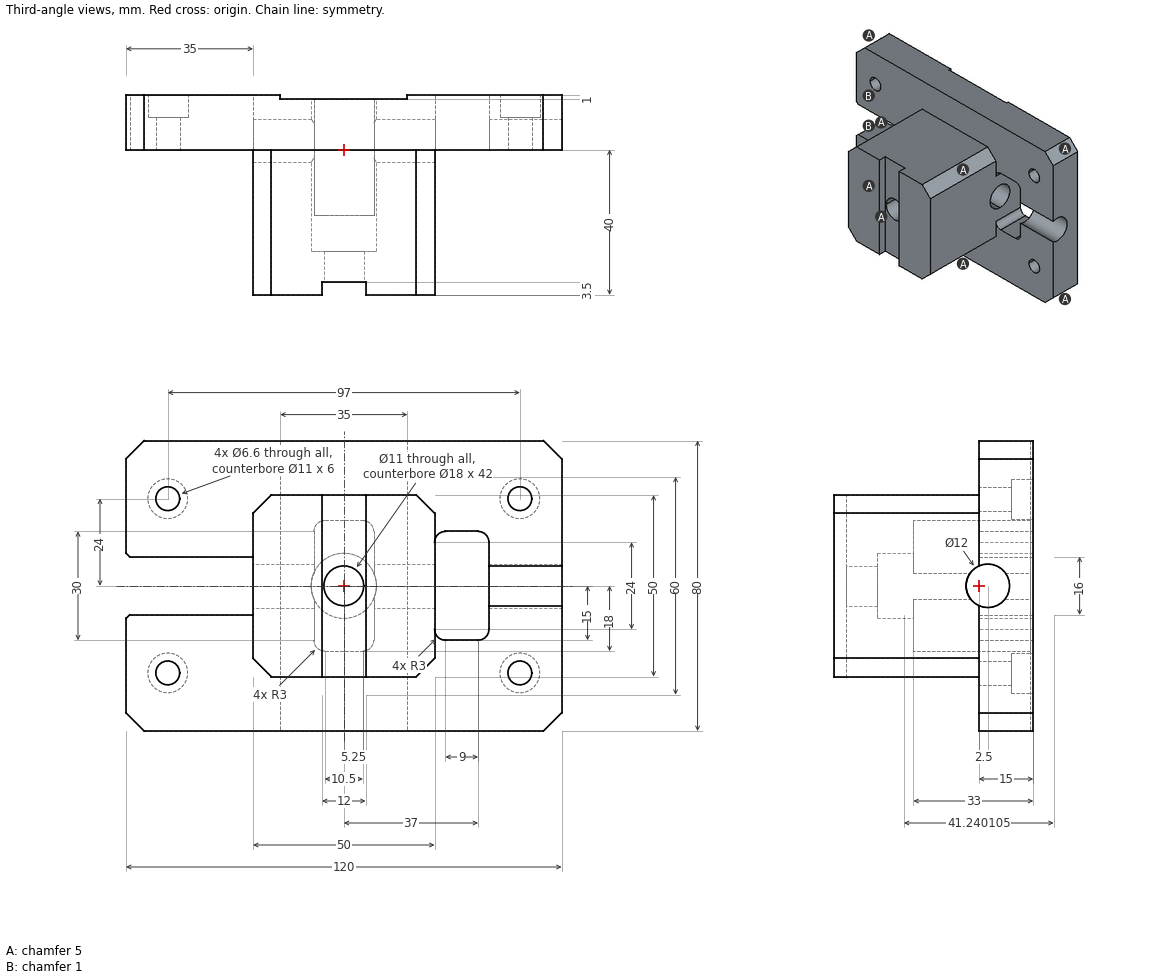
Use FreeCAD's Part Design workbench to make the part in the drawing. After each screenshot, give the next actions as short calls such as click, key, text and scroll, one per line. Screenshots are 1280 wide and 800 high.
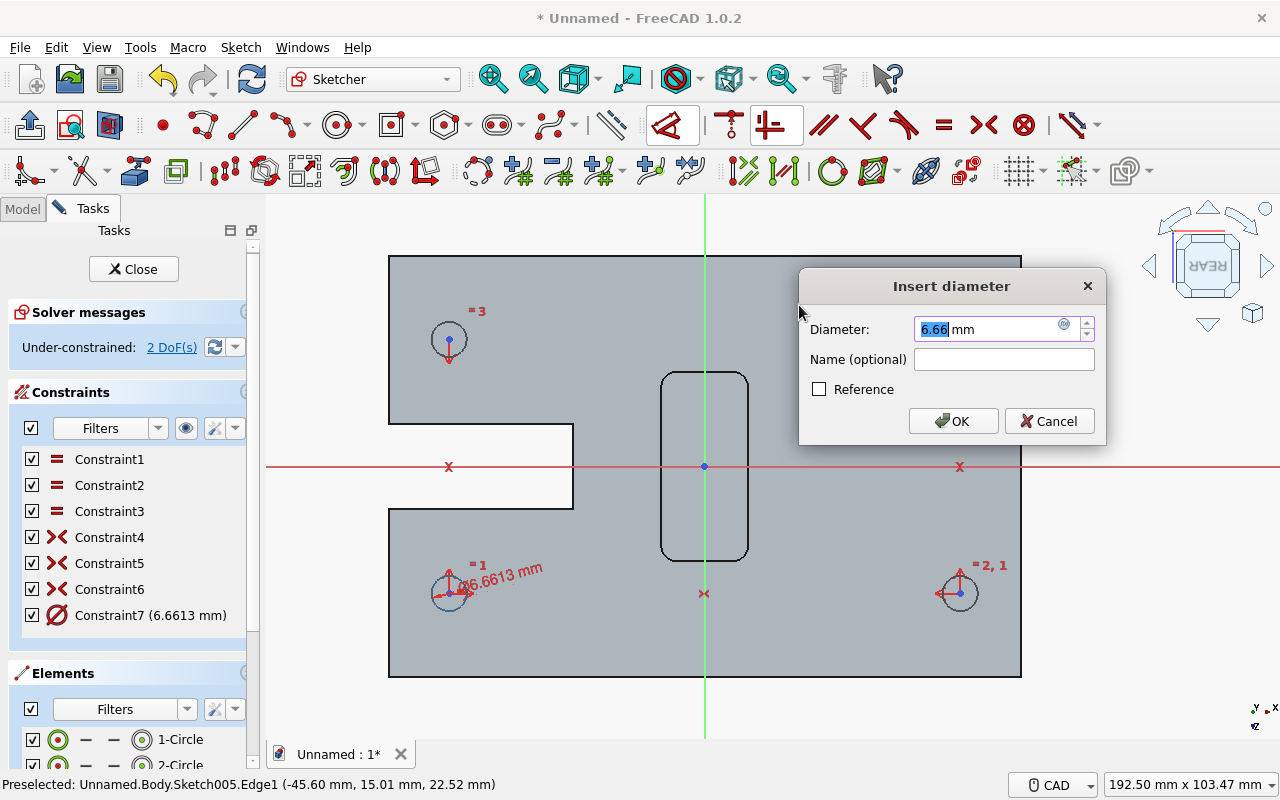
text(6.6)
key(Return)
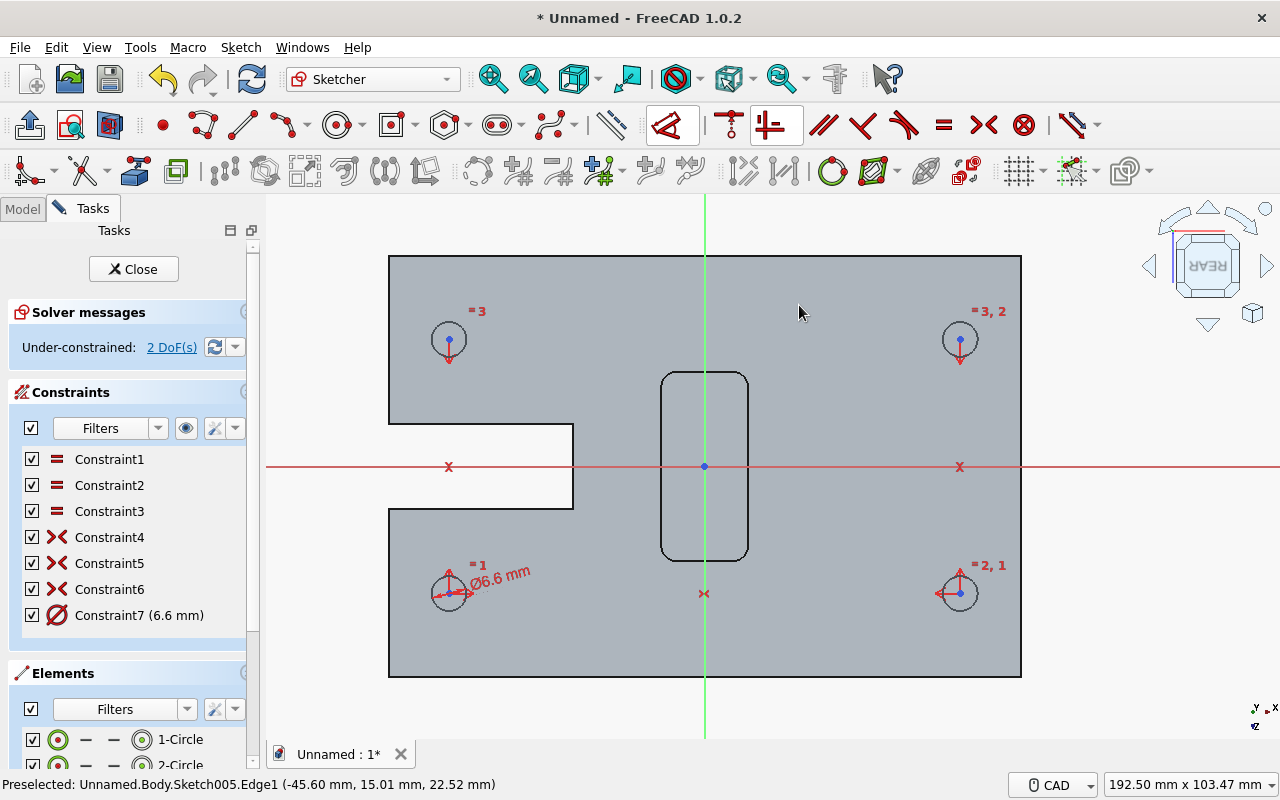
click(449, 594)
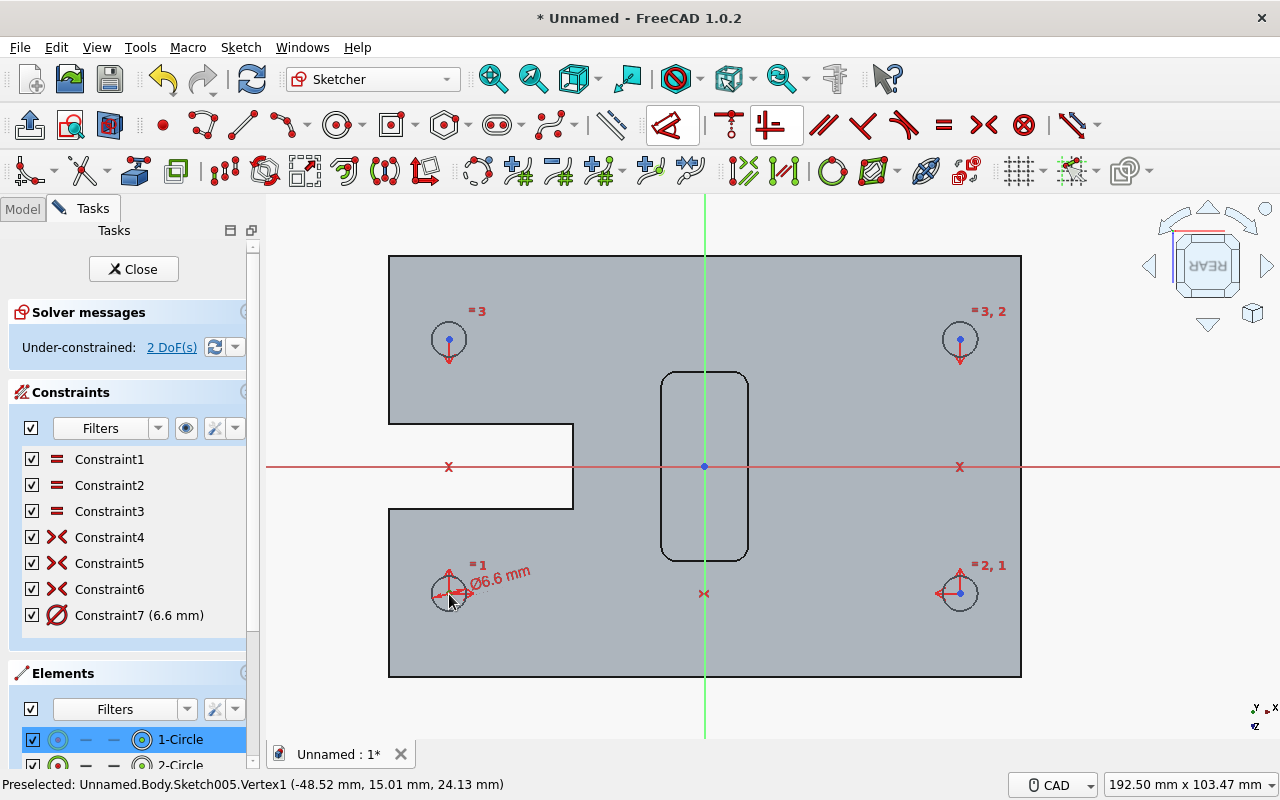
key(i)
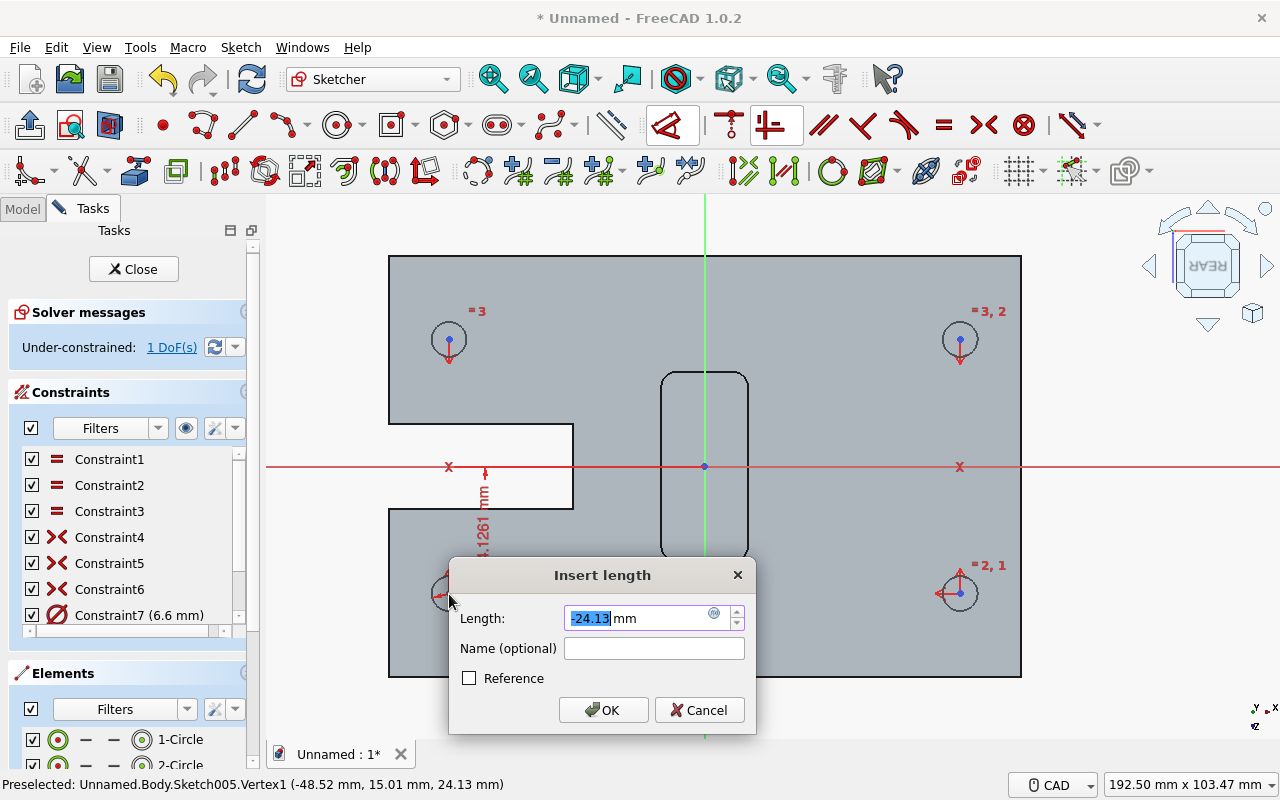
text(-24)
key(Return)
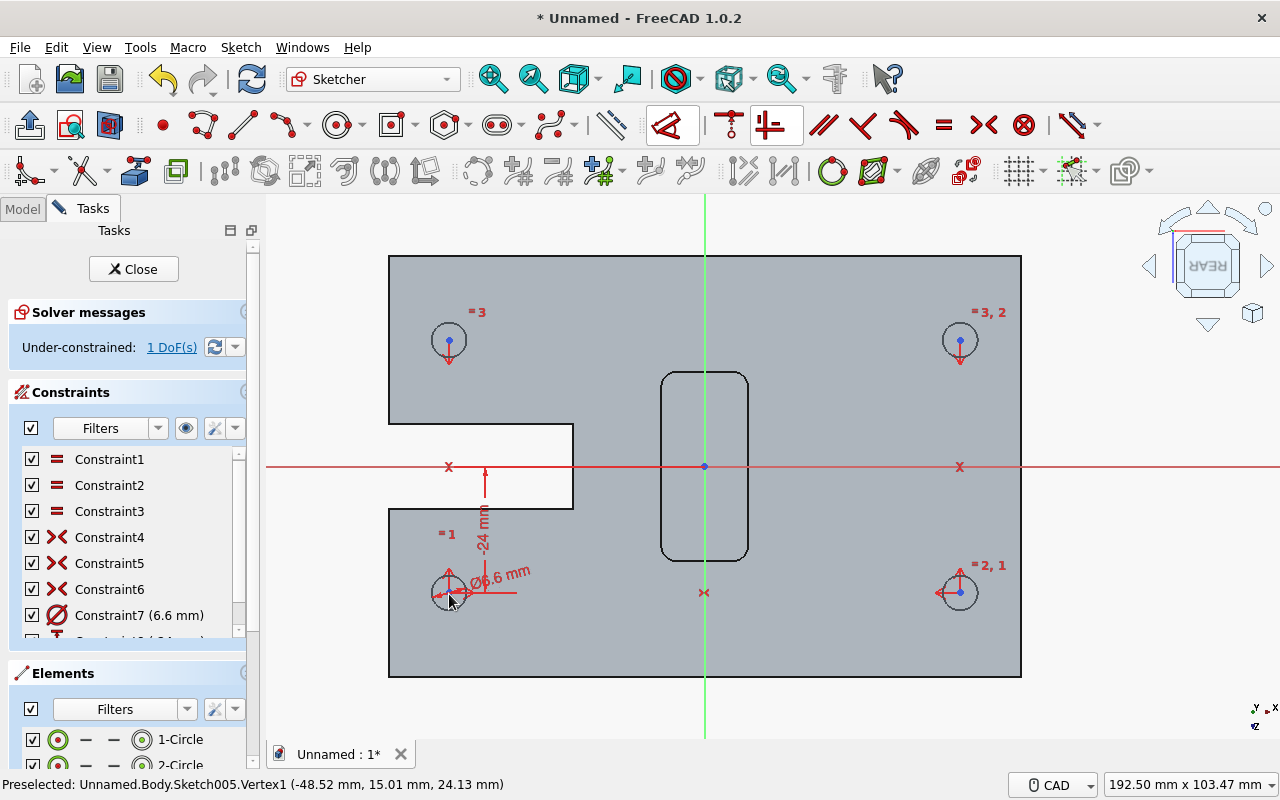
click(449, 593)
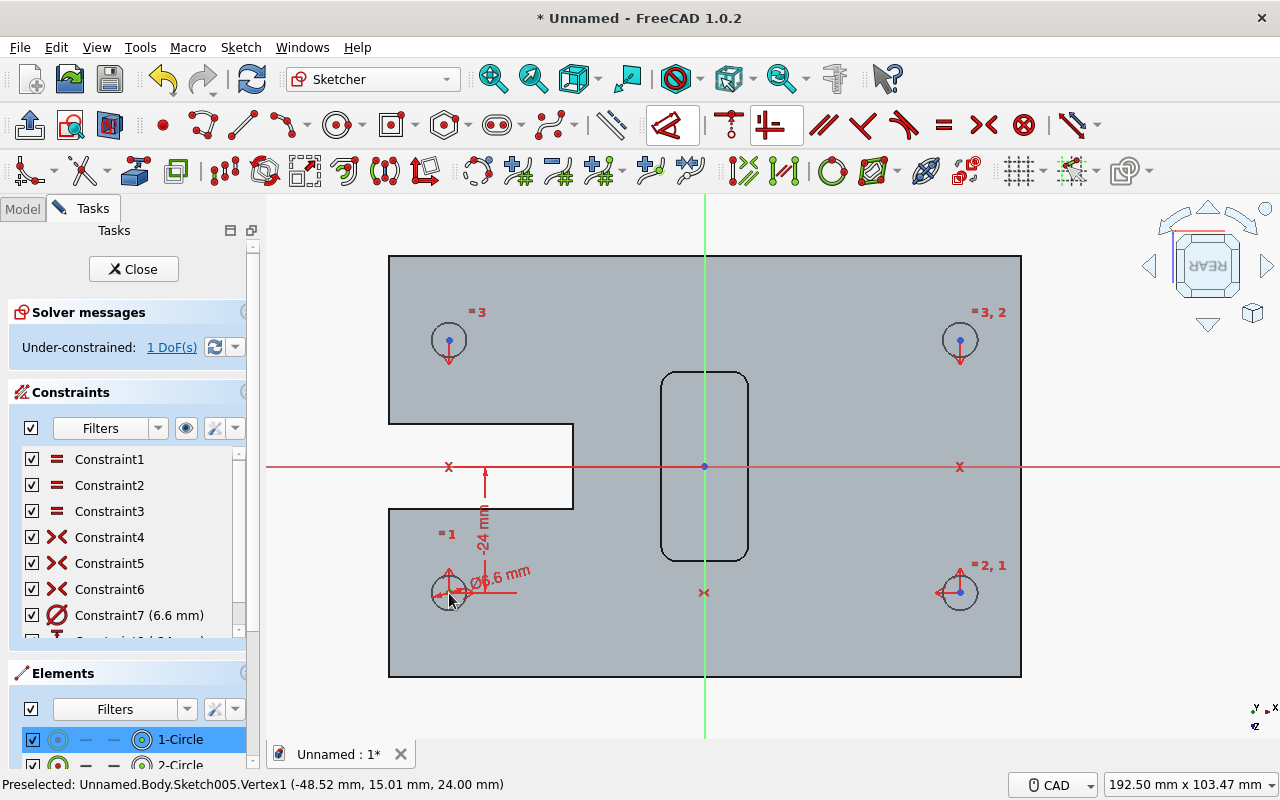
click(960, 593)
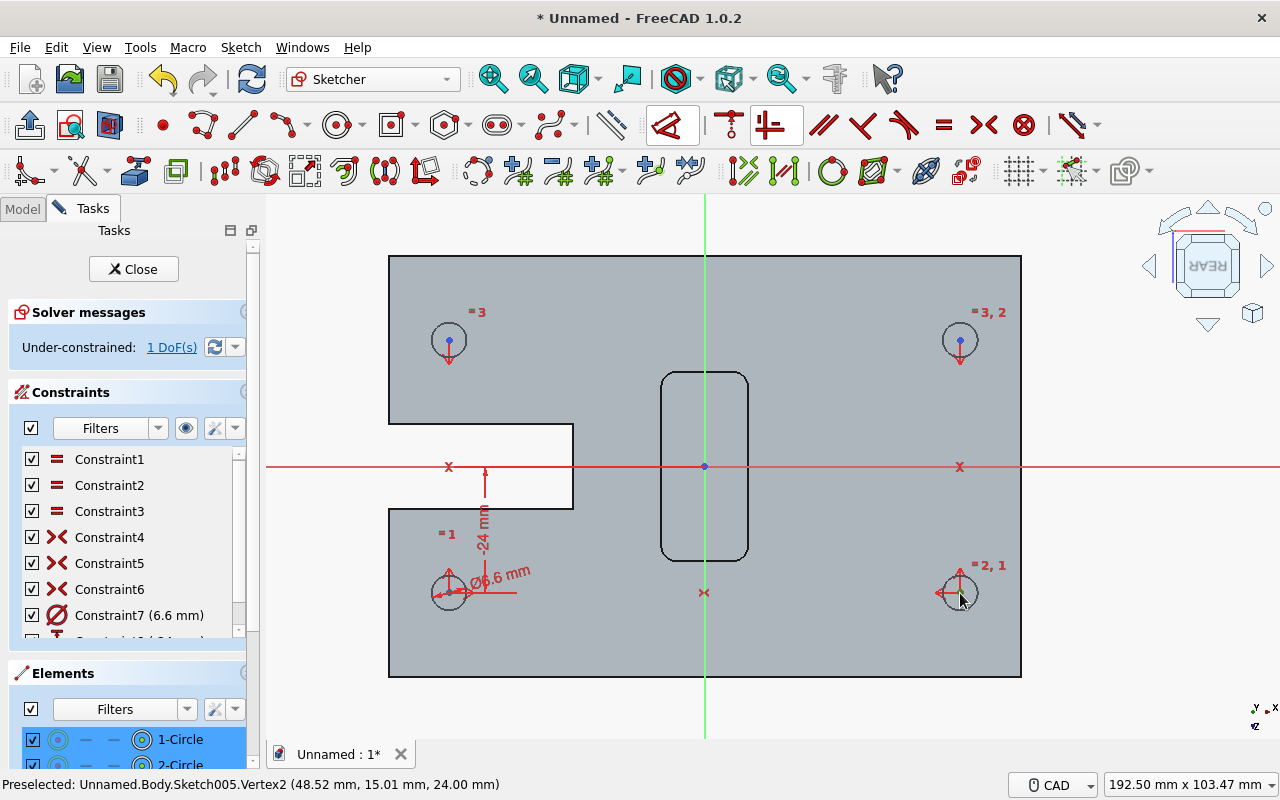
key(l)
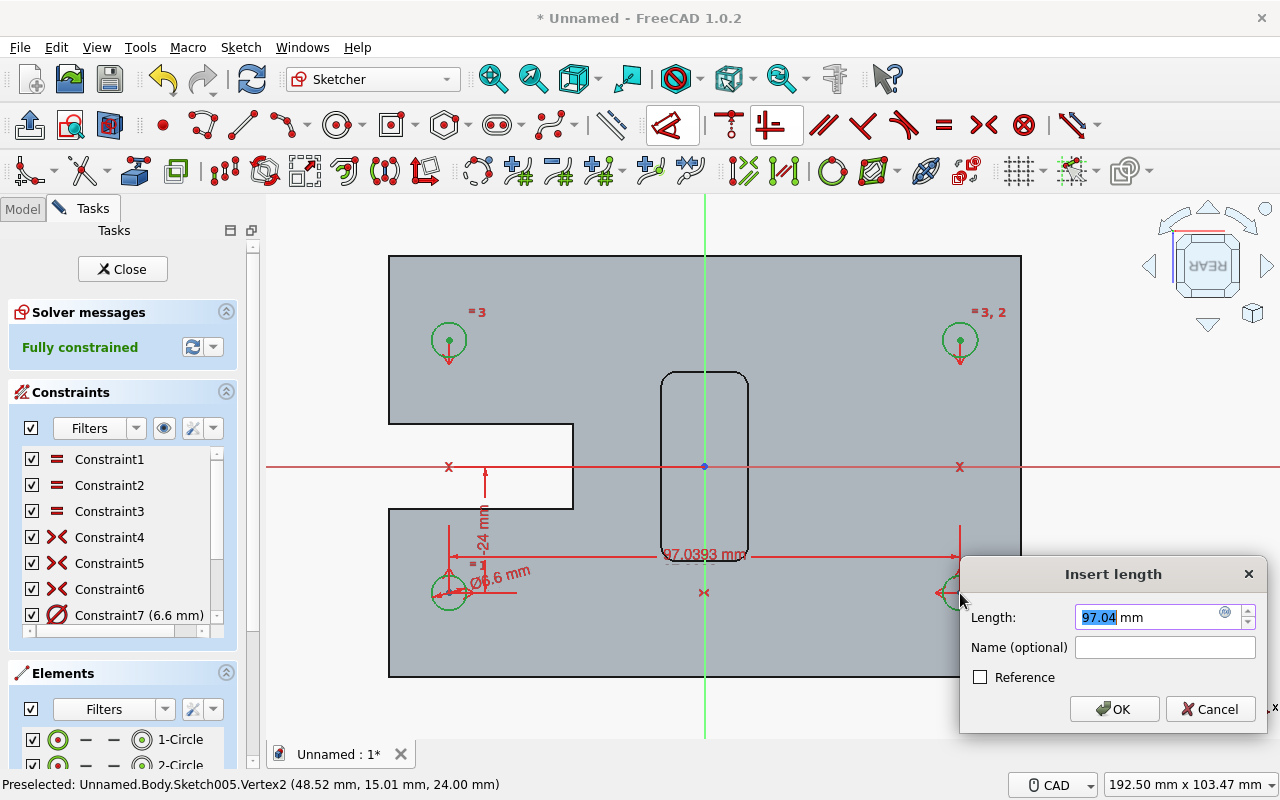
text(97)
key(Return)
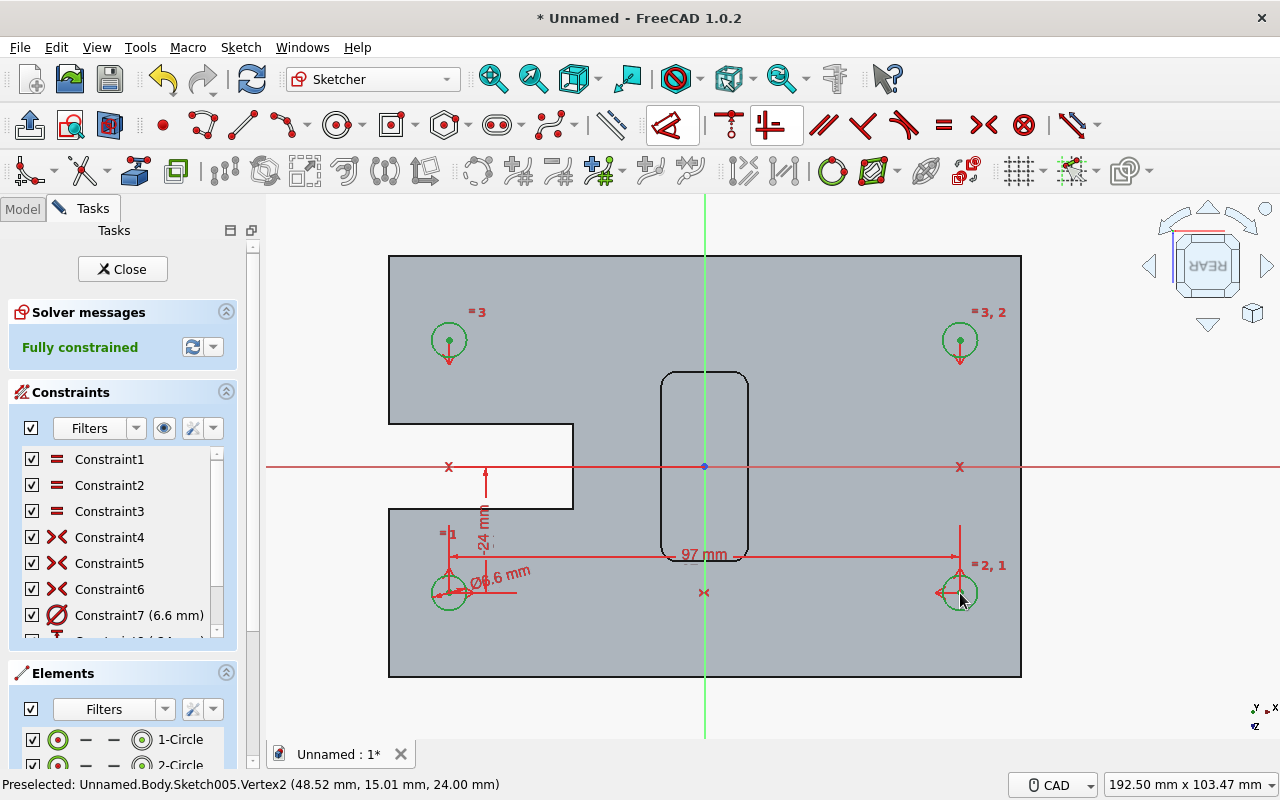
click(123, 269)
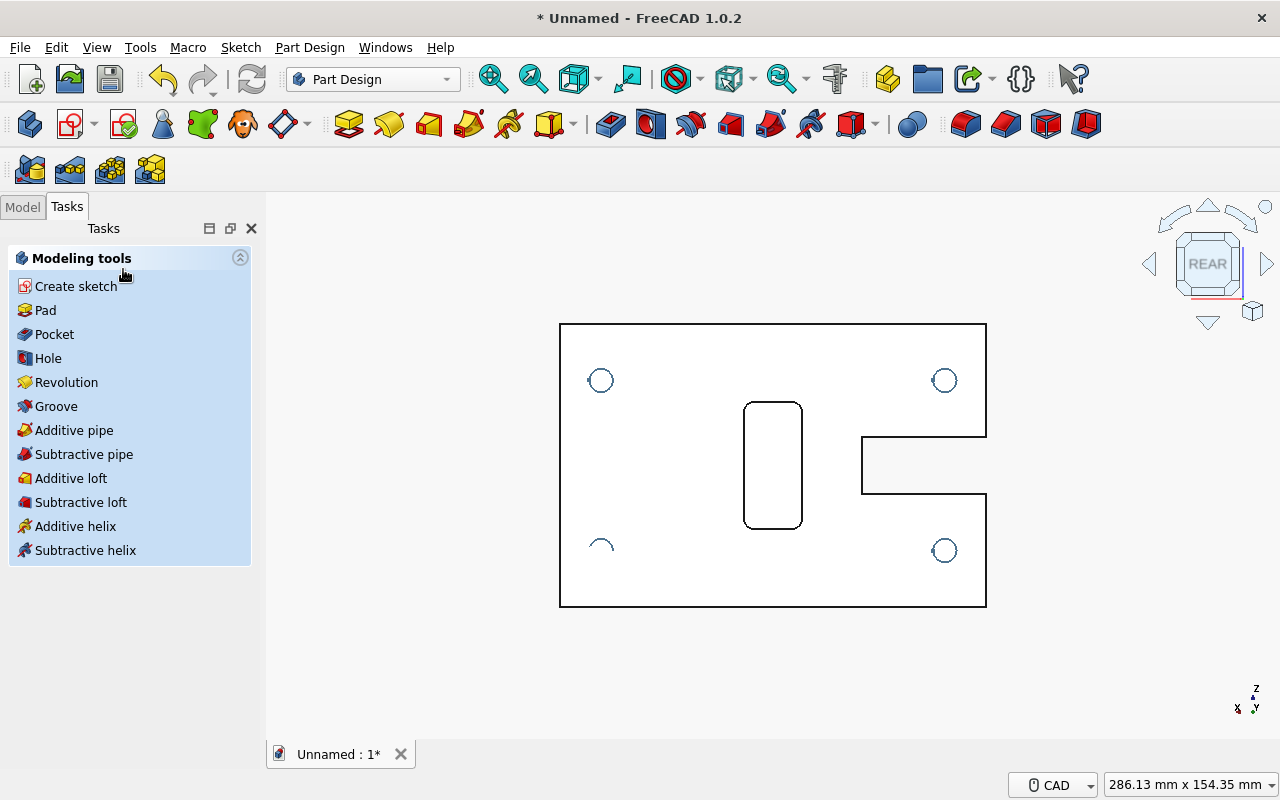
click(652, 124)